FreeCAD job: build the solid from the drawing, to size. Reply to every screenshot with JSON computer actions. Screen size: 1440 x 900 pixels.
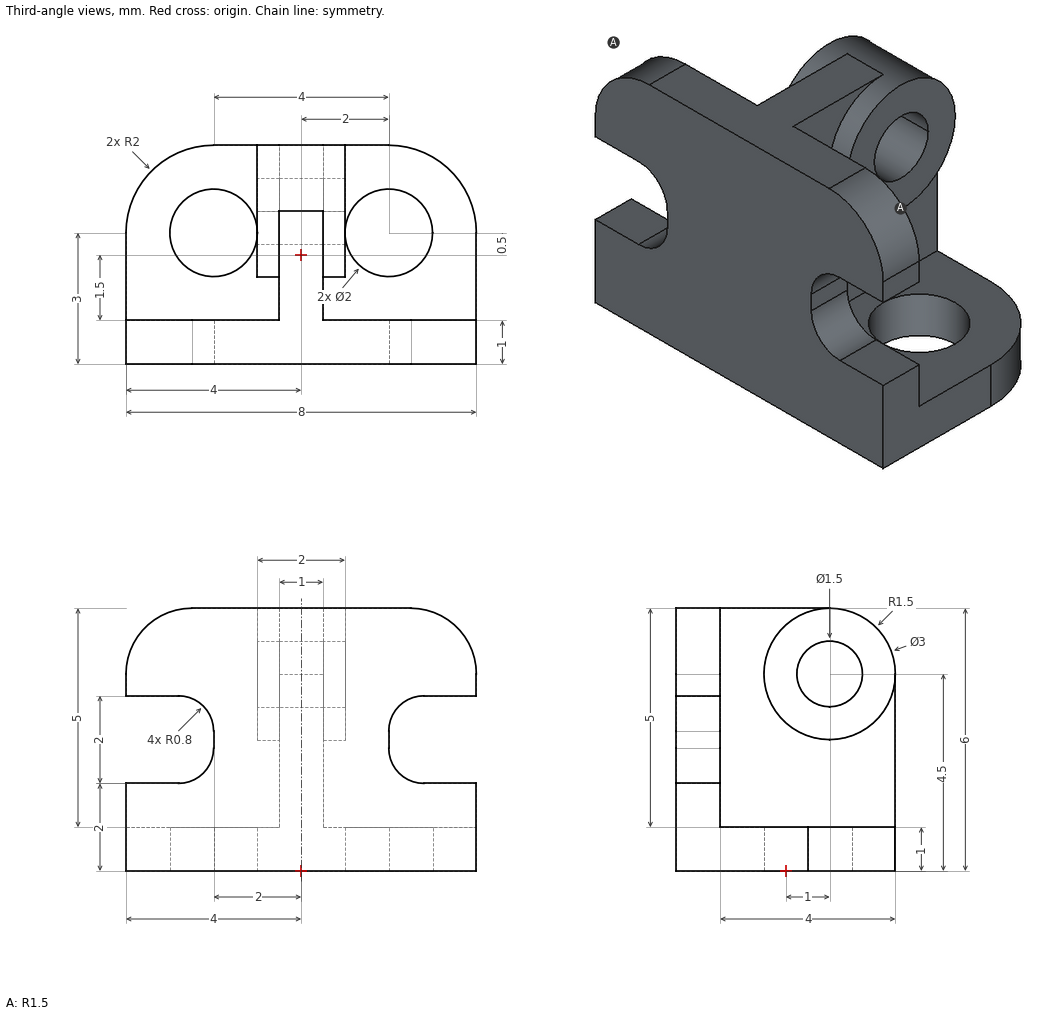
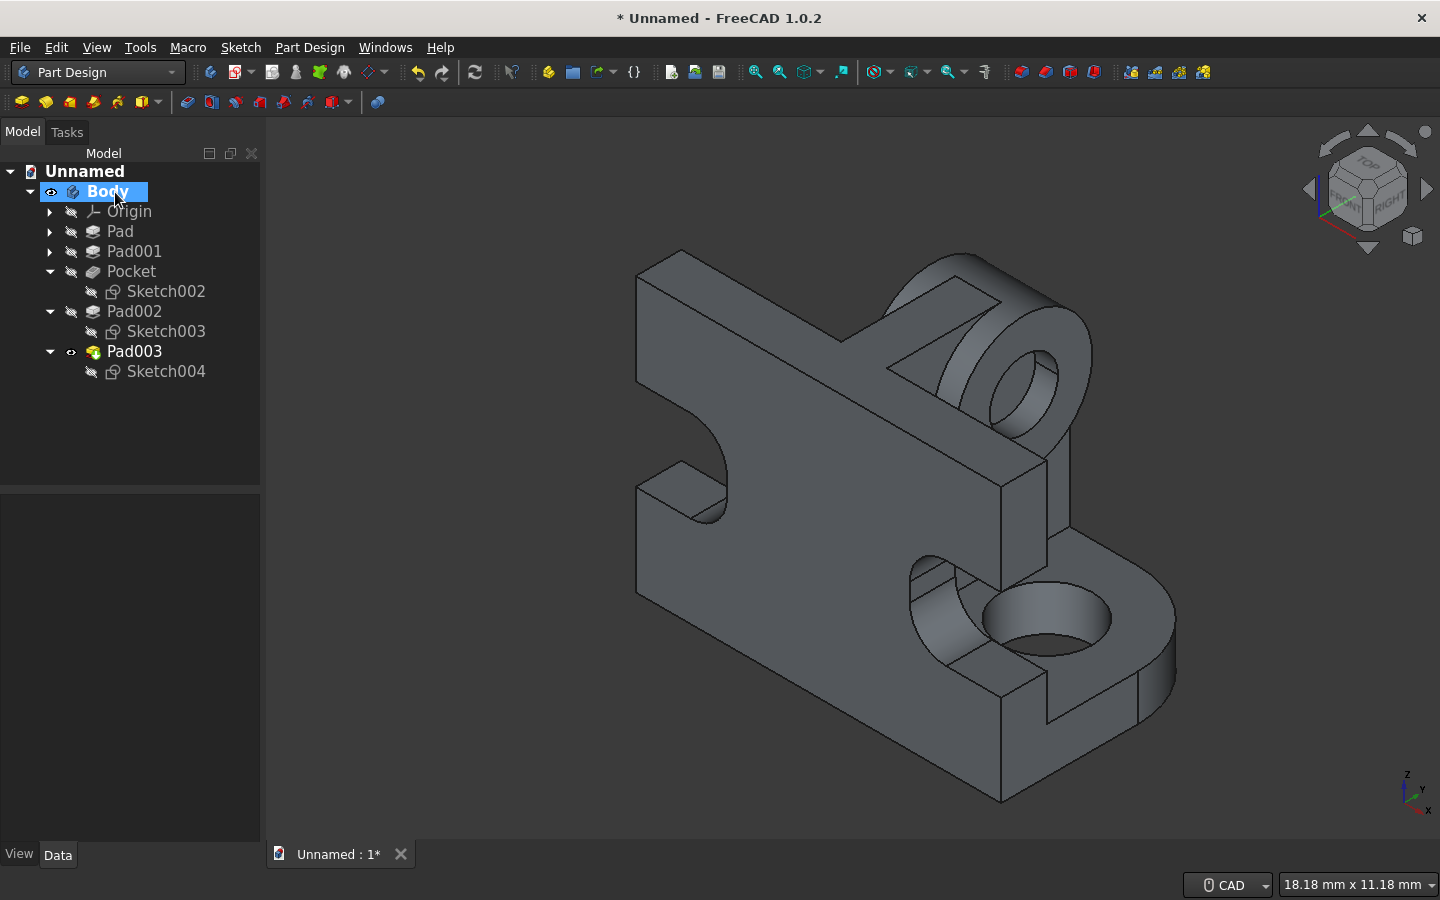
{"action": "key", "text": "3"}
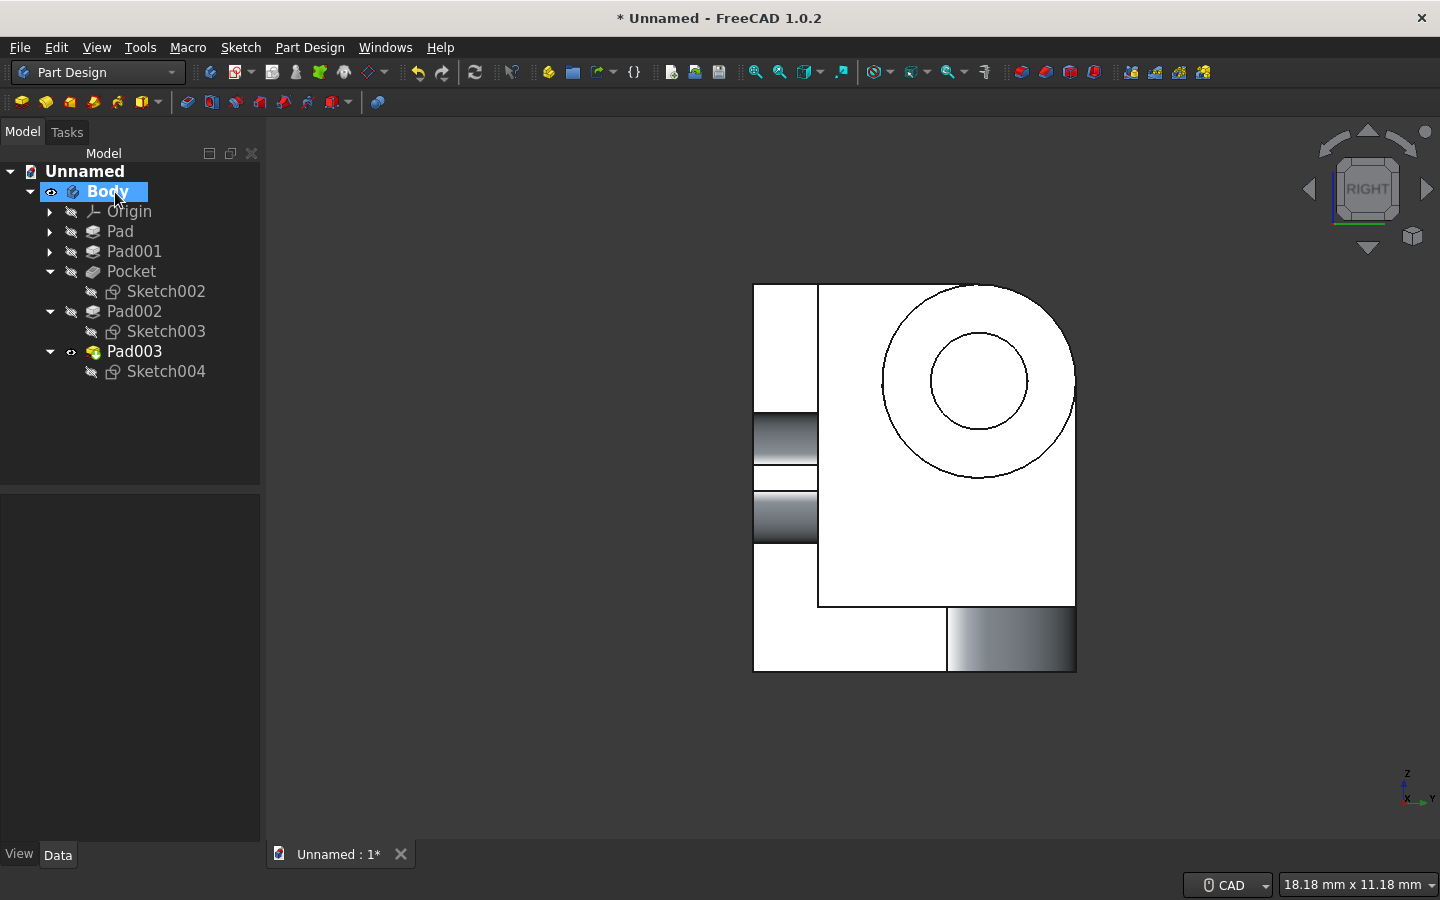
{"action": "left_click", "coordinate": [910, 537]}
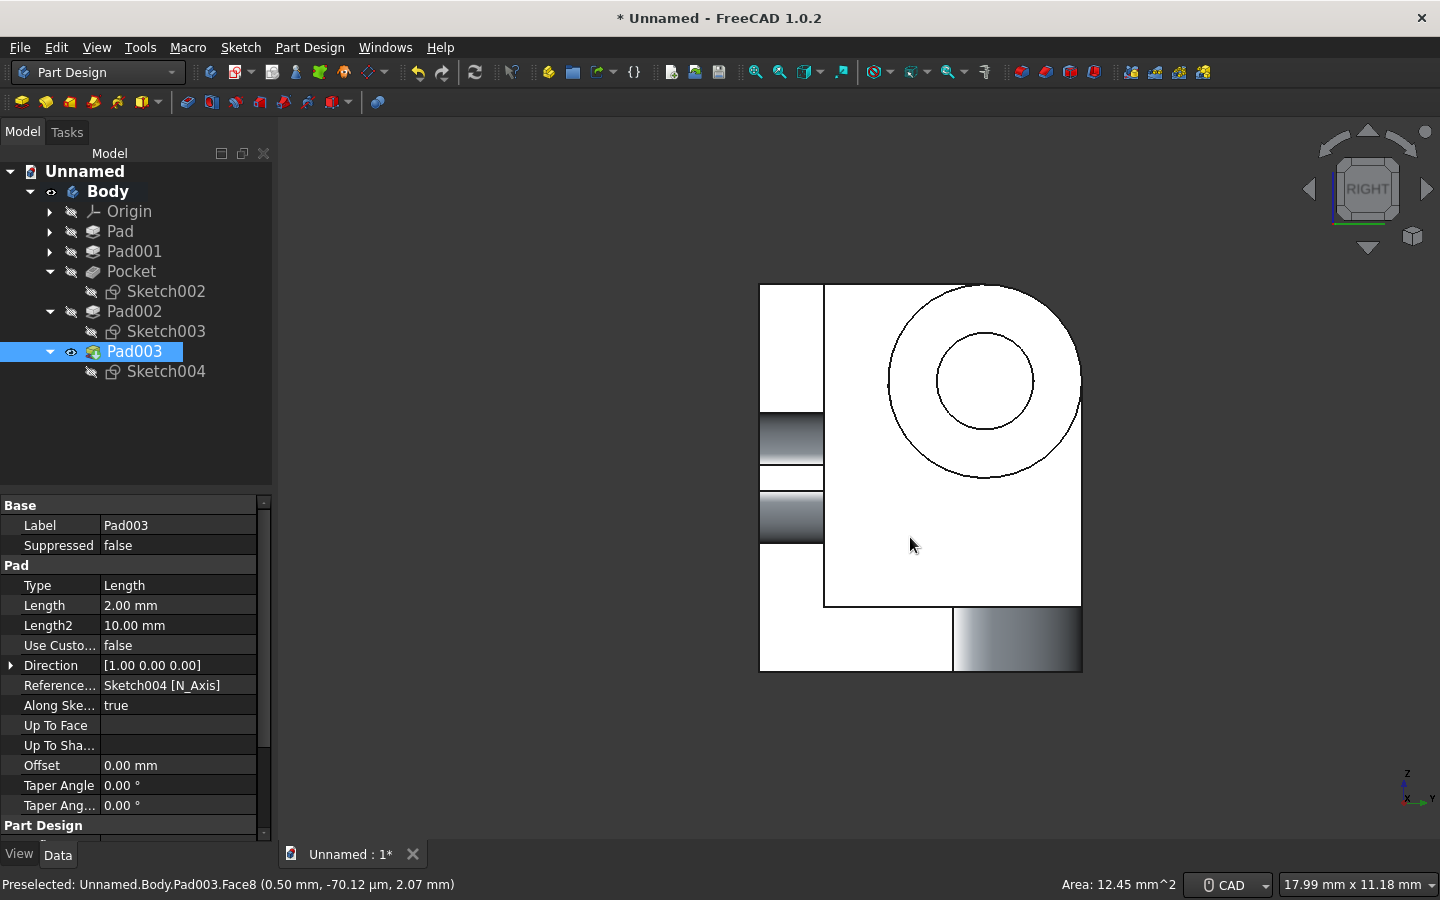
{"action": "left_click", "coordinate": [236, 72]}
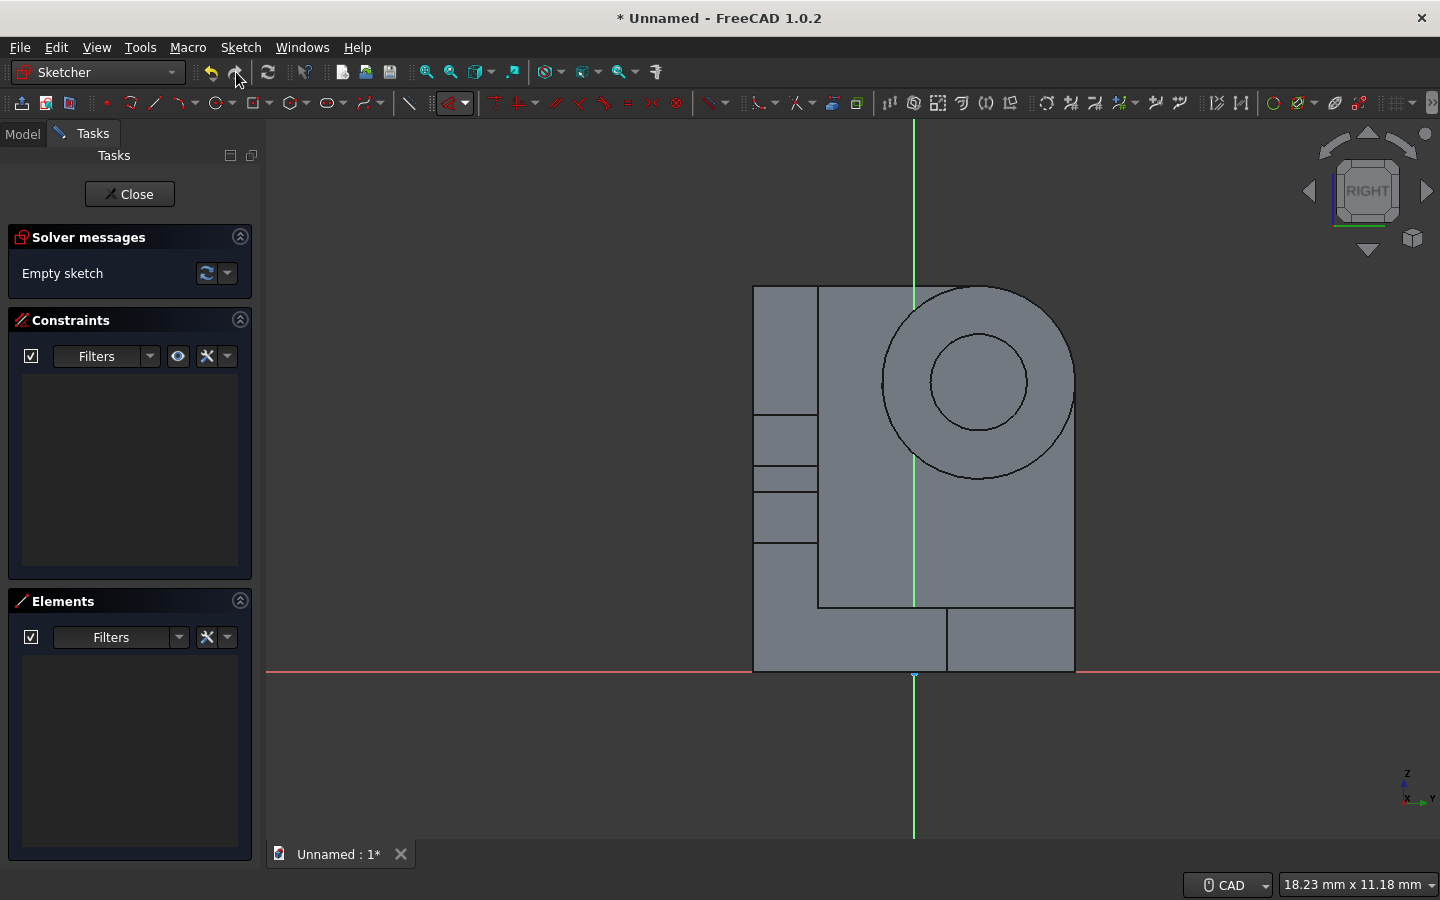
{"action": "scroll", "coordinate": [1028, 358], "scroll_direction": "up", "scroll_amount": 8}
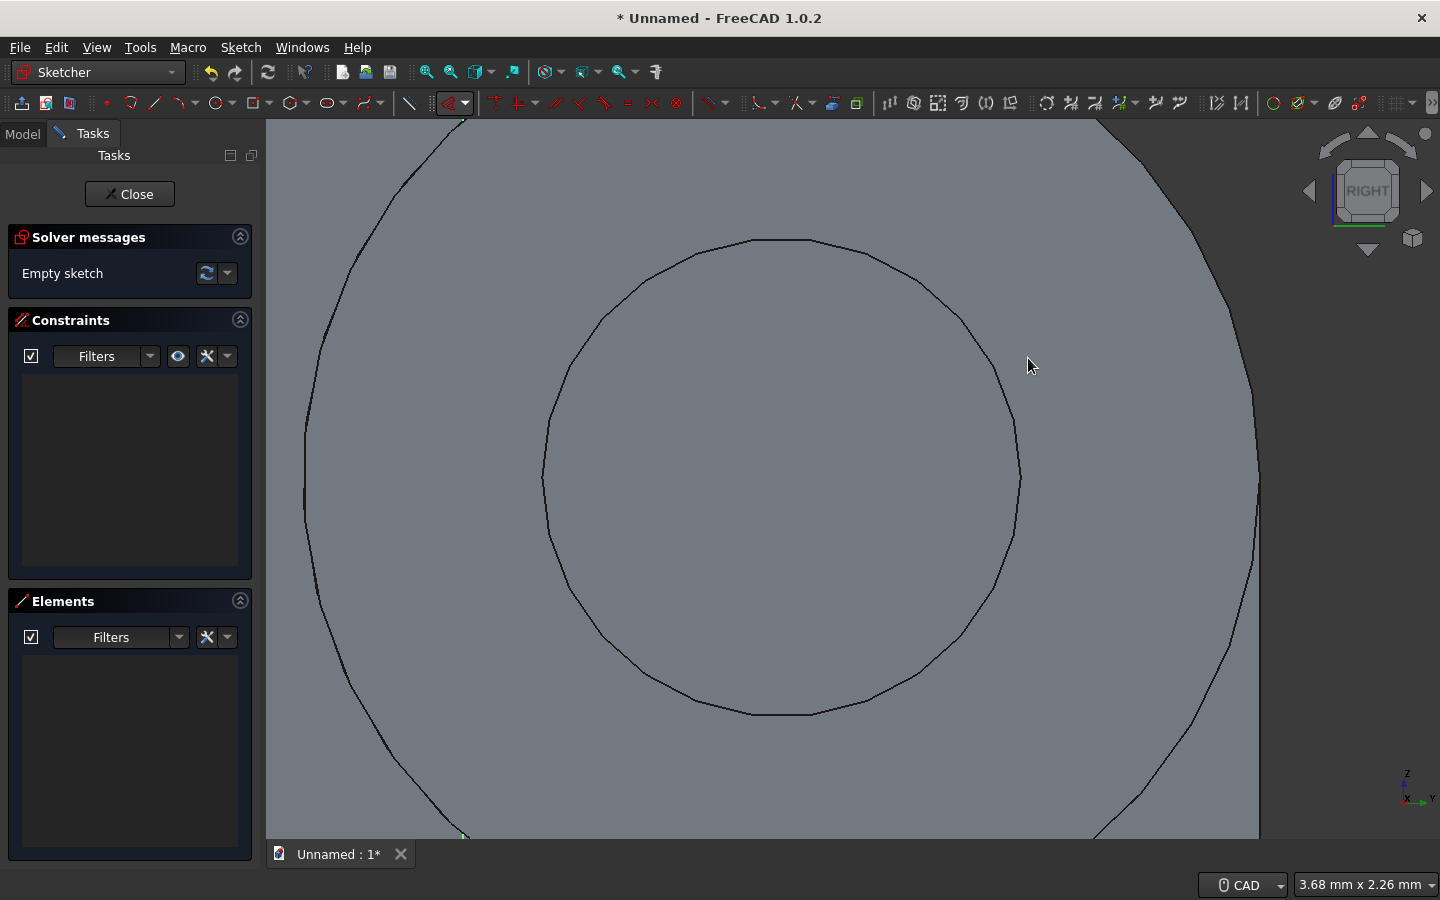
{"action": "left_click", "coordinate": [216, 104]}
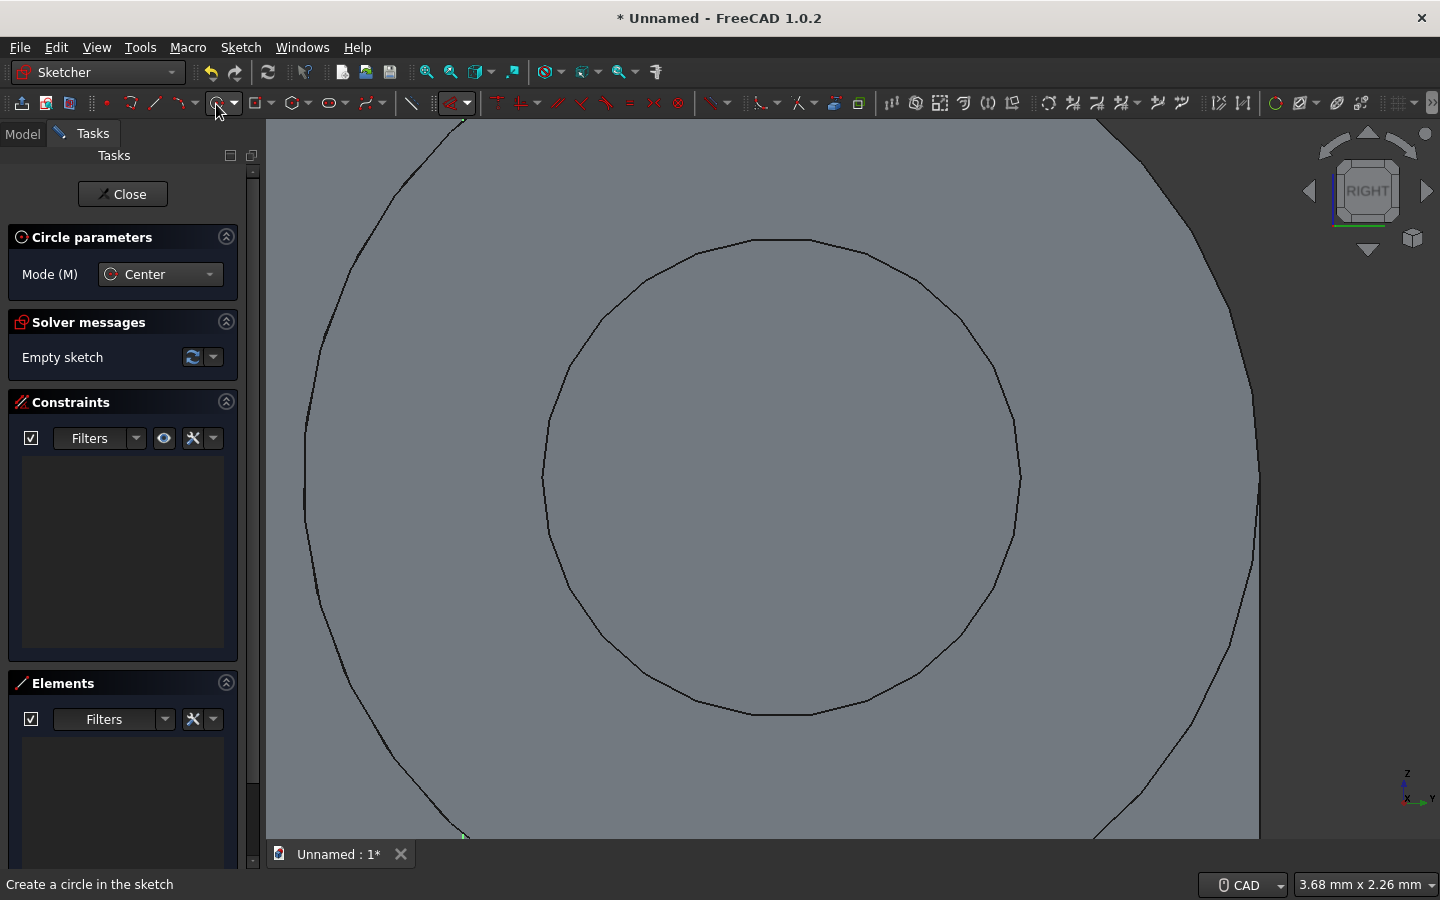
{"action": "left_click", "coordinate": [782, 478]}
{"action": "mouse_move", "coordinate": [951, 308]}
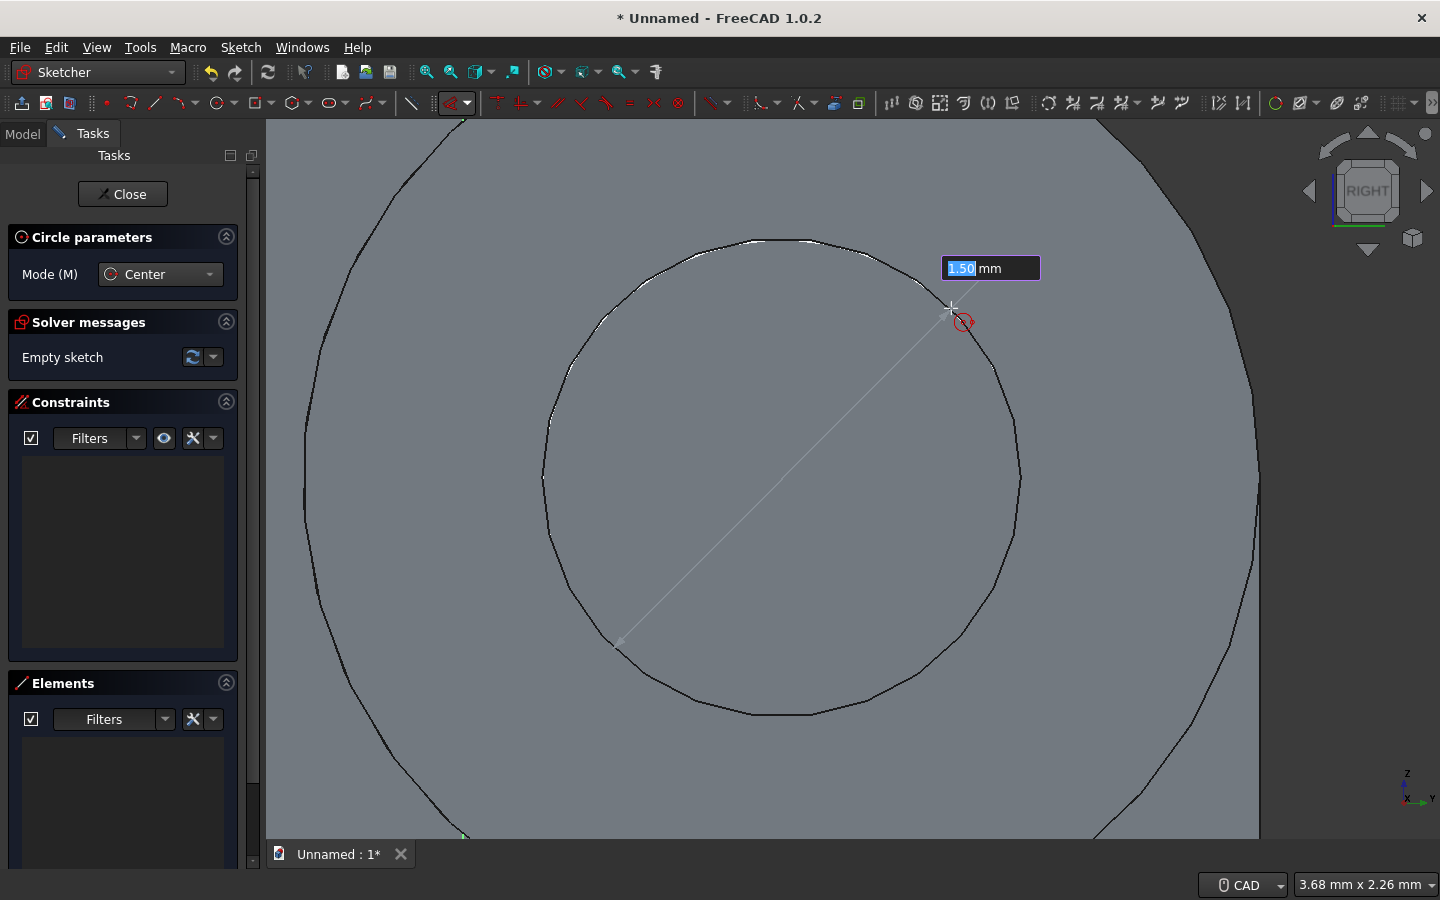
{"action": "type", "text": "1.5"}
{"action": "key", "text": "Return"}
{"action": "key", "text": "Escape"}